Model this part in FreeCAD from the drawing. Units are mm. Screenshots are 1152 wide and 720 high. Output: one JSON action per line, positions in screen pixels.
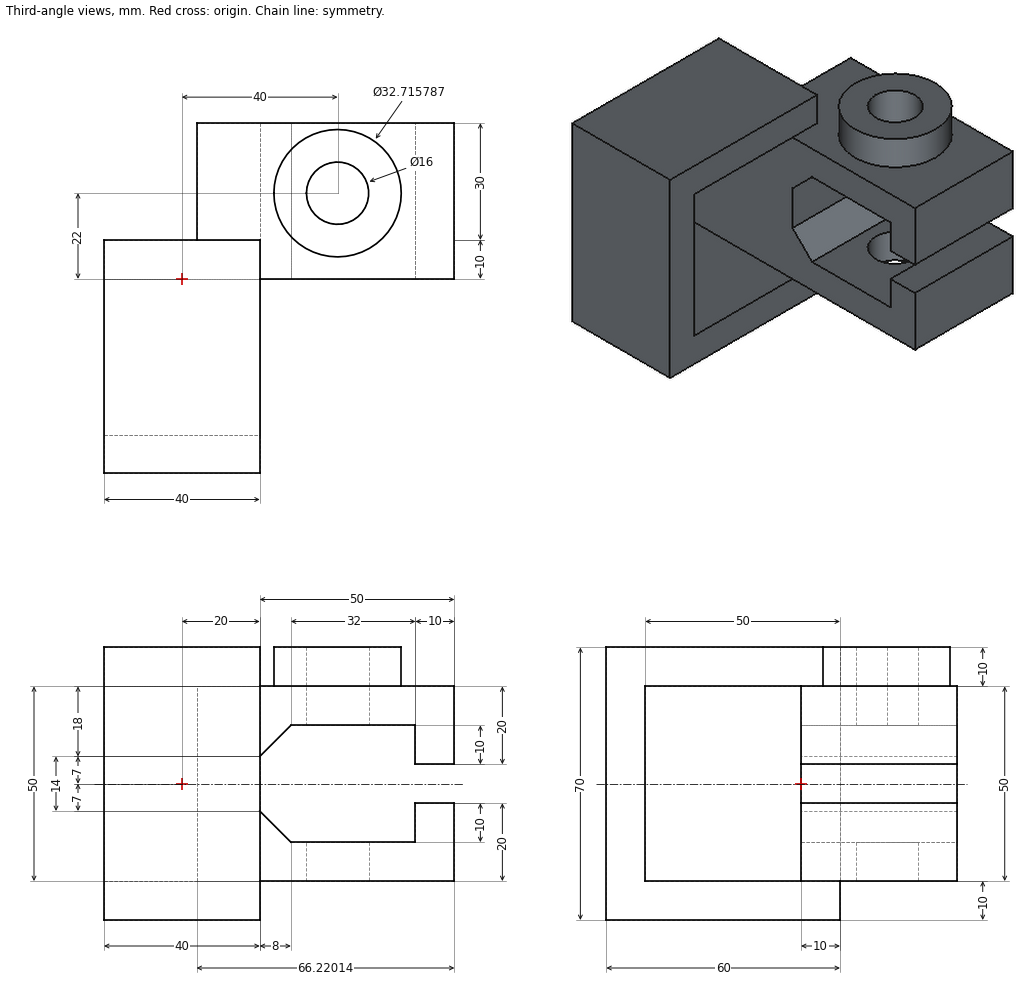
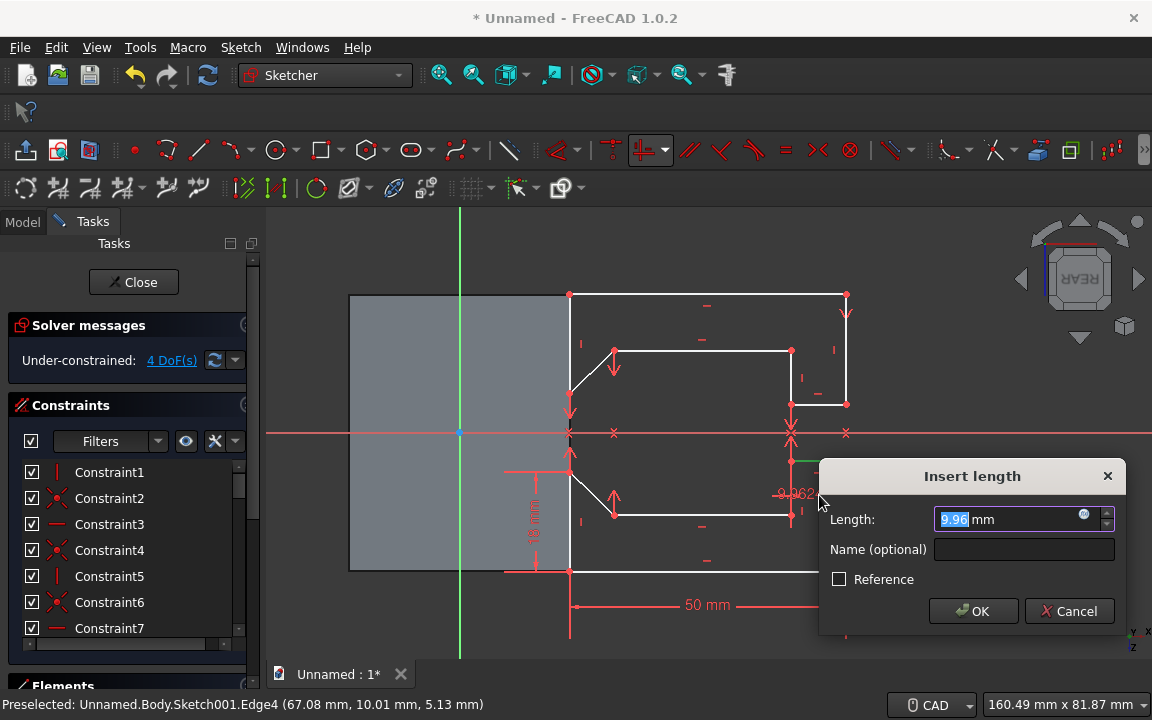
{"action": "type", "text": "10"}
{"action": "key", "text": "Return"}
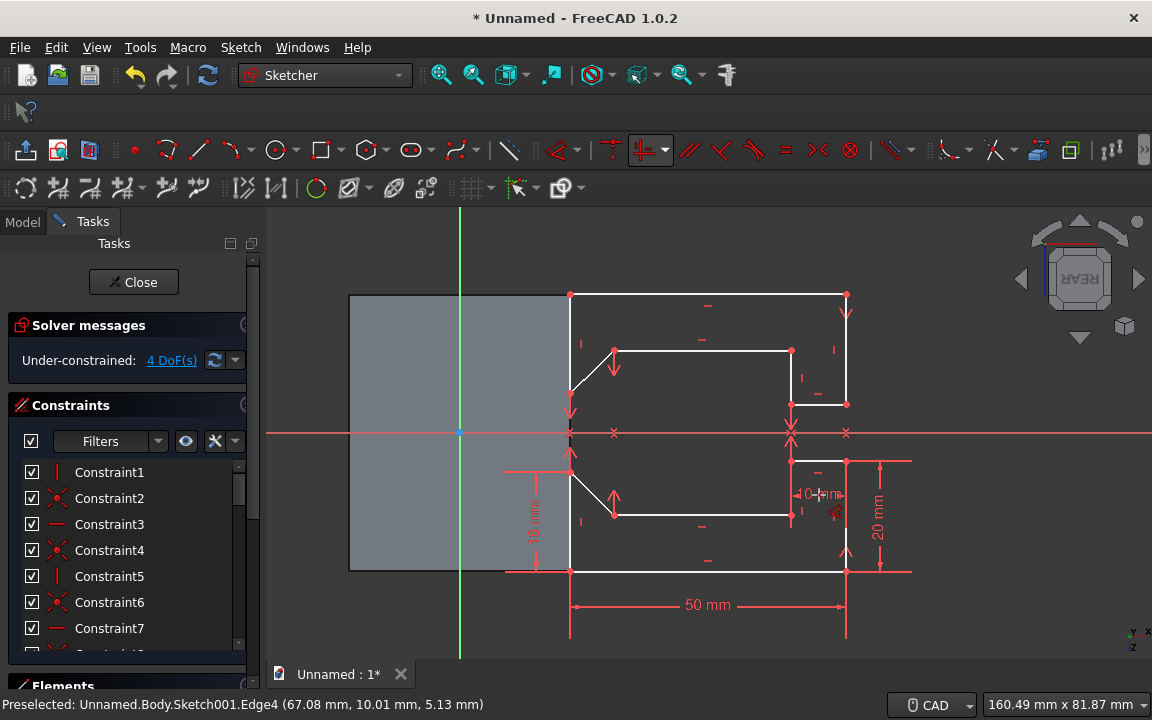
{"action": "left_click", "coordinate": [791, 477]}
{"action": "left_click", "coordinate": [757, 469]}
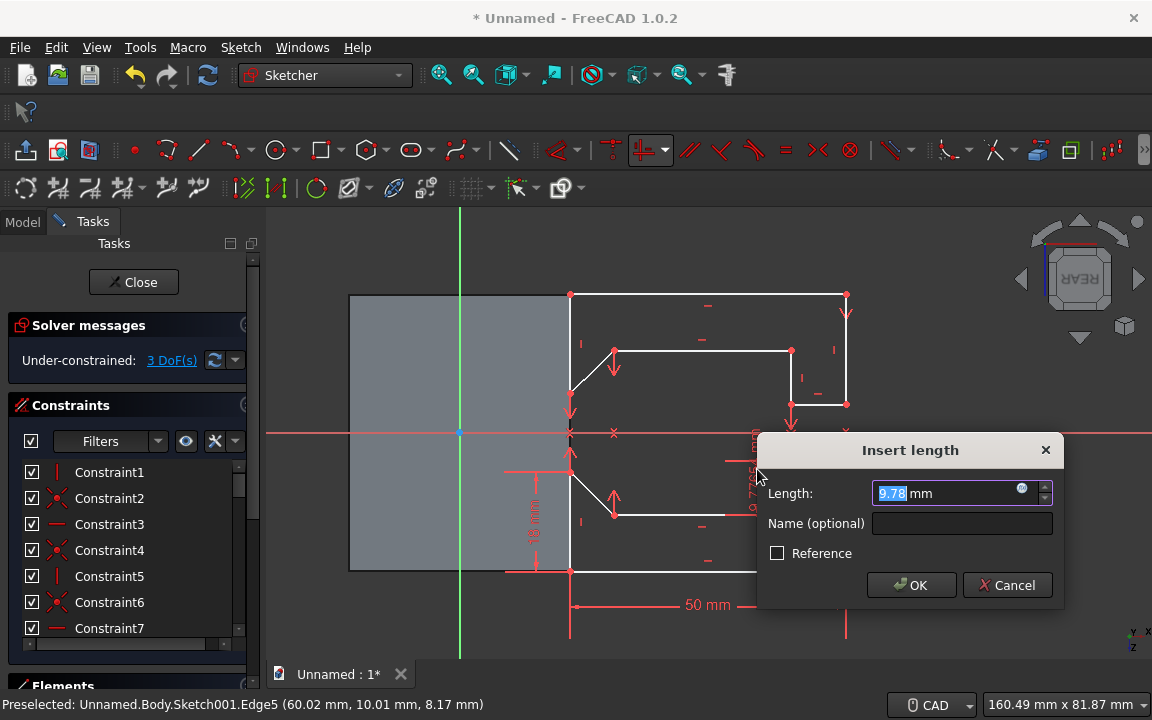
{"action": "type", "text": "10"}
{"action": "key", "text": "Return"}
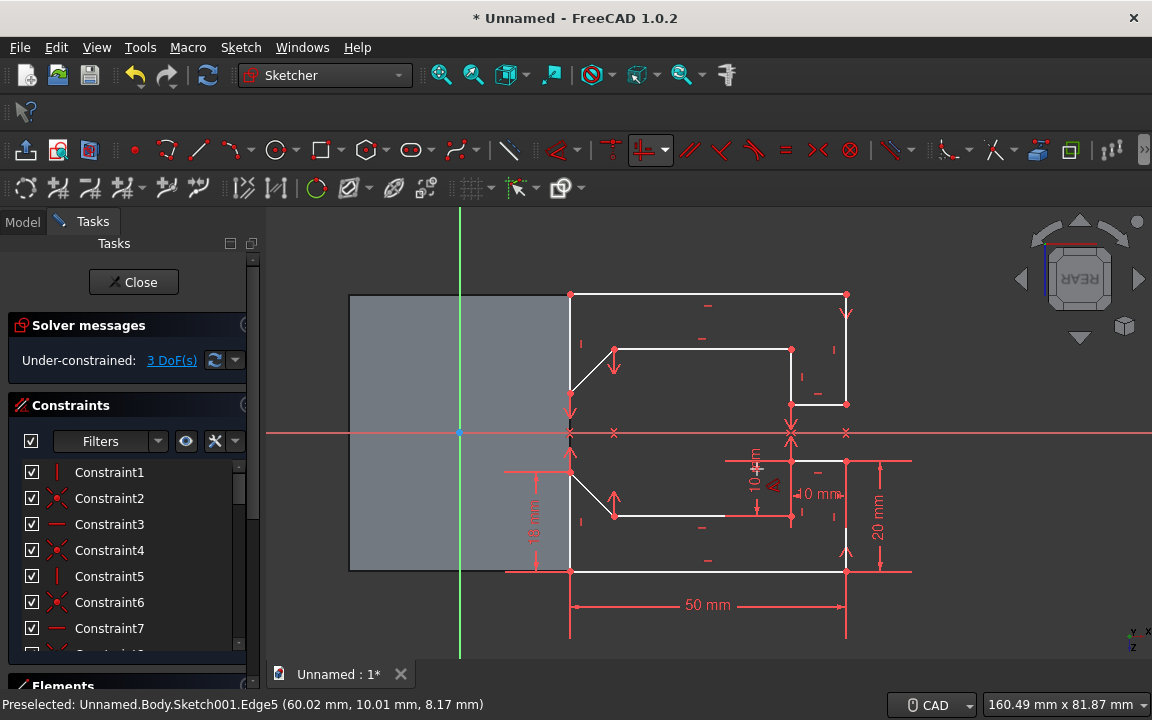
{"action": "left_click", "coordinate": [738, 516]}
{"action": "left_click", "coordinate": [703, 550]}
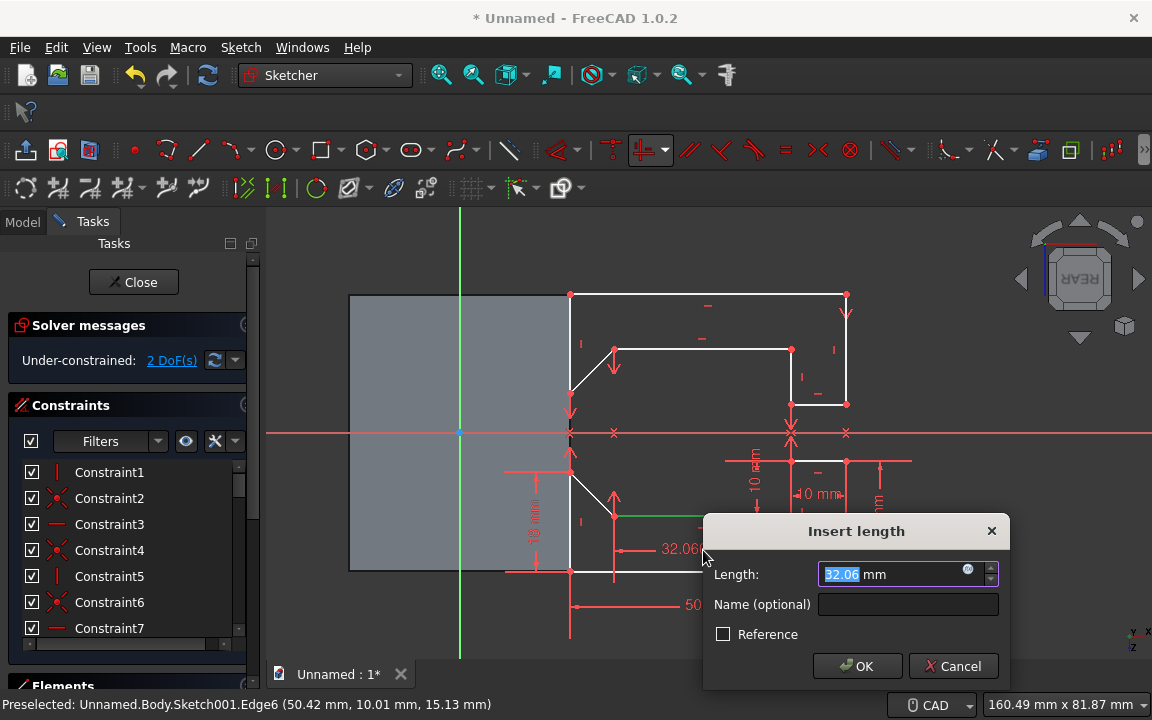
{"action": "type", "text": "32"}
{"action": "key", "text": "Return"}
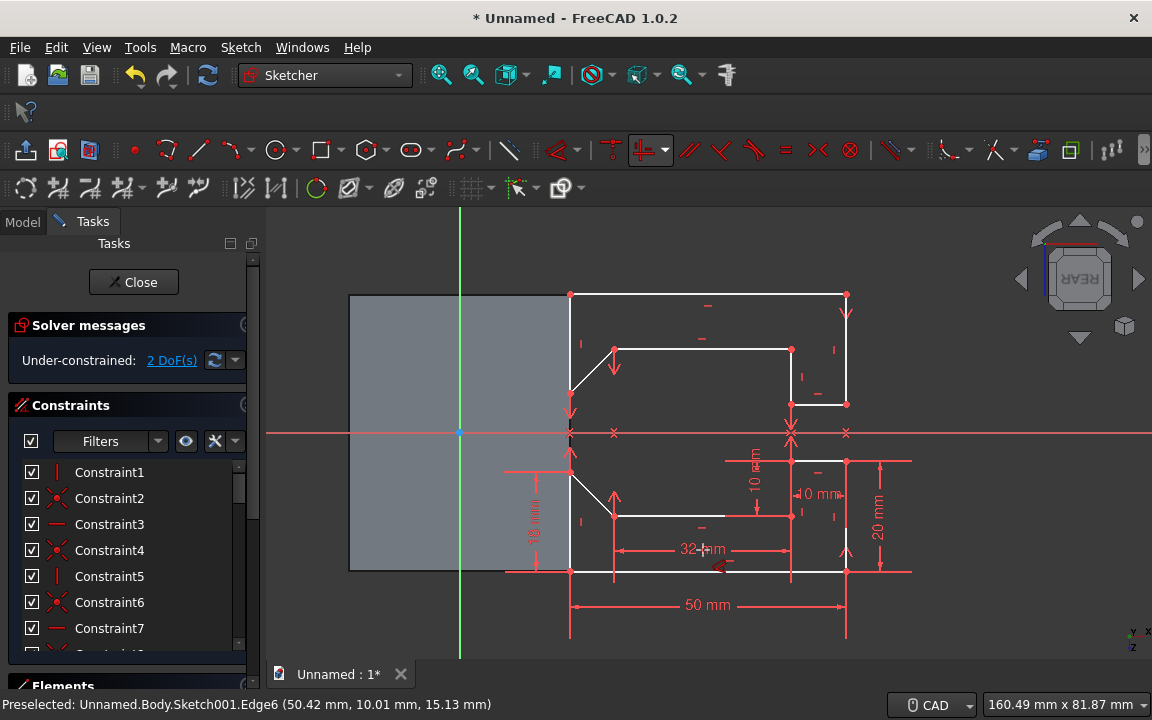
{"action": "left_click", "coordinate": [570, 472]}
{"action": "left_click", "coordinate": [426, 453]}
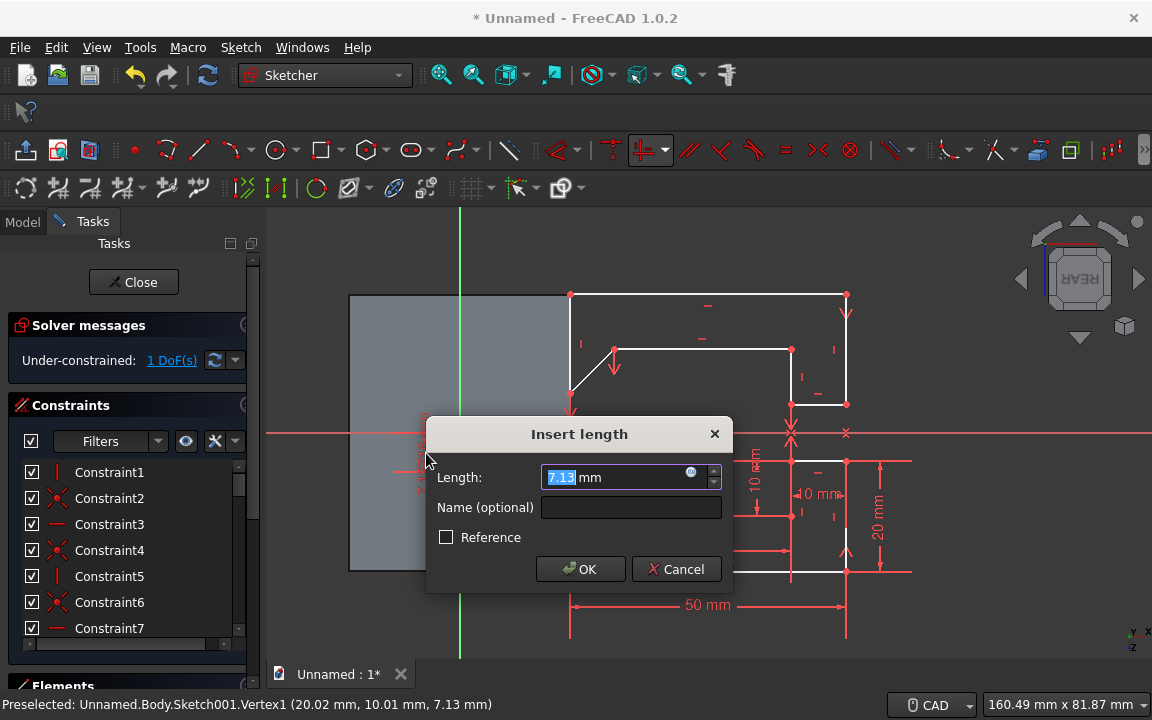
{"action": "type", "text": "7"}
{"action": "key", "text": "Return"}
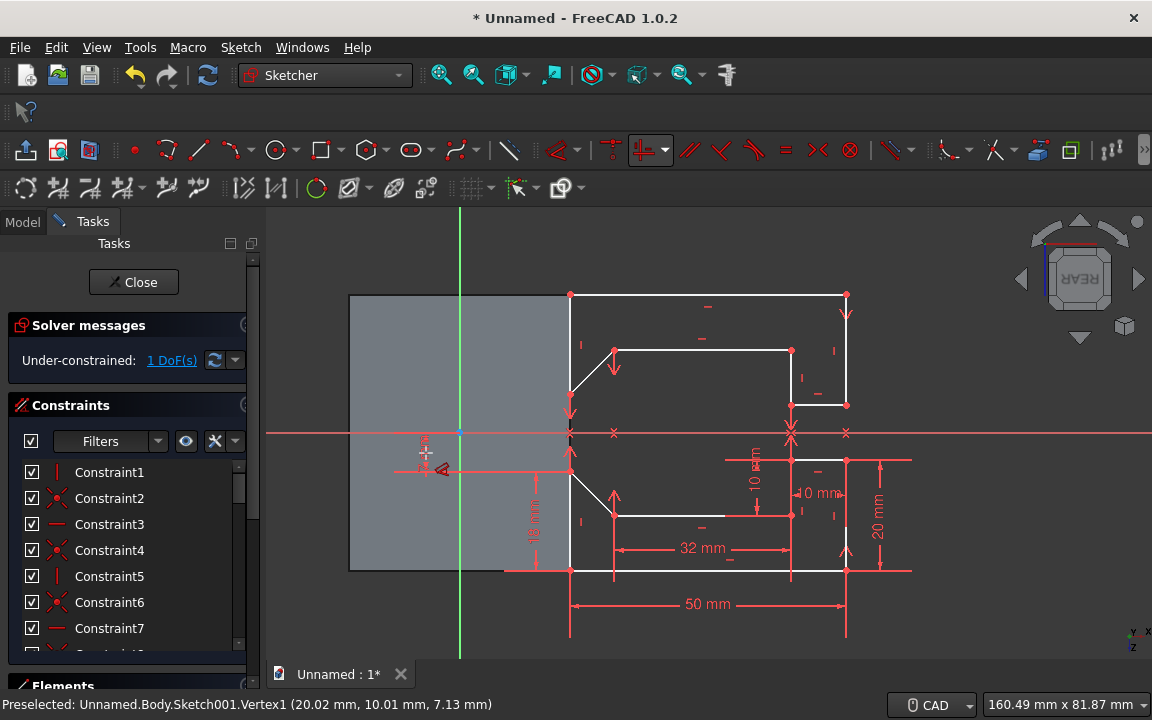
{"action": "left_click", "coordinate": [570, 472]}
{"action": "left_click", "coordinate": [515, 399]}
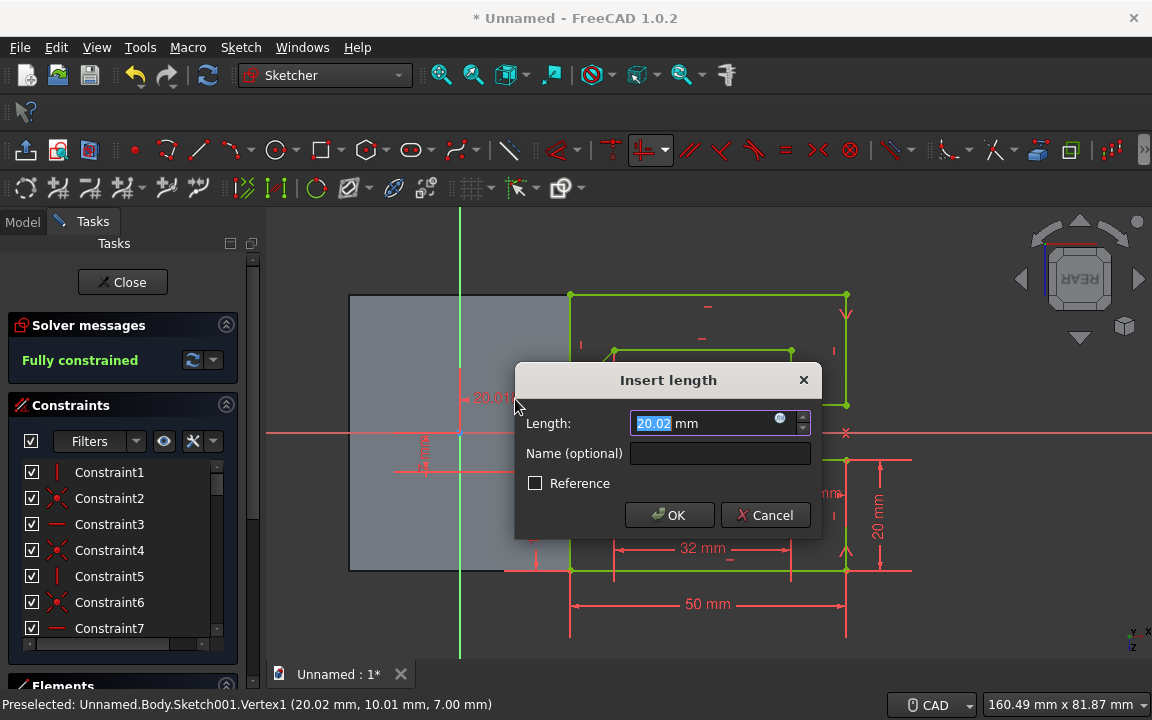
{"action": "type", "text": "20"}
{"action": "key", "text": "Return"}
{"action": "key", "text": "Escape"}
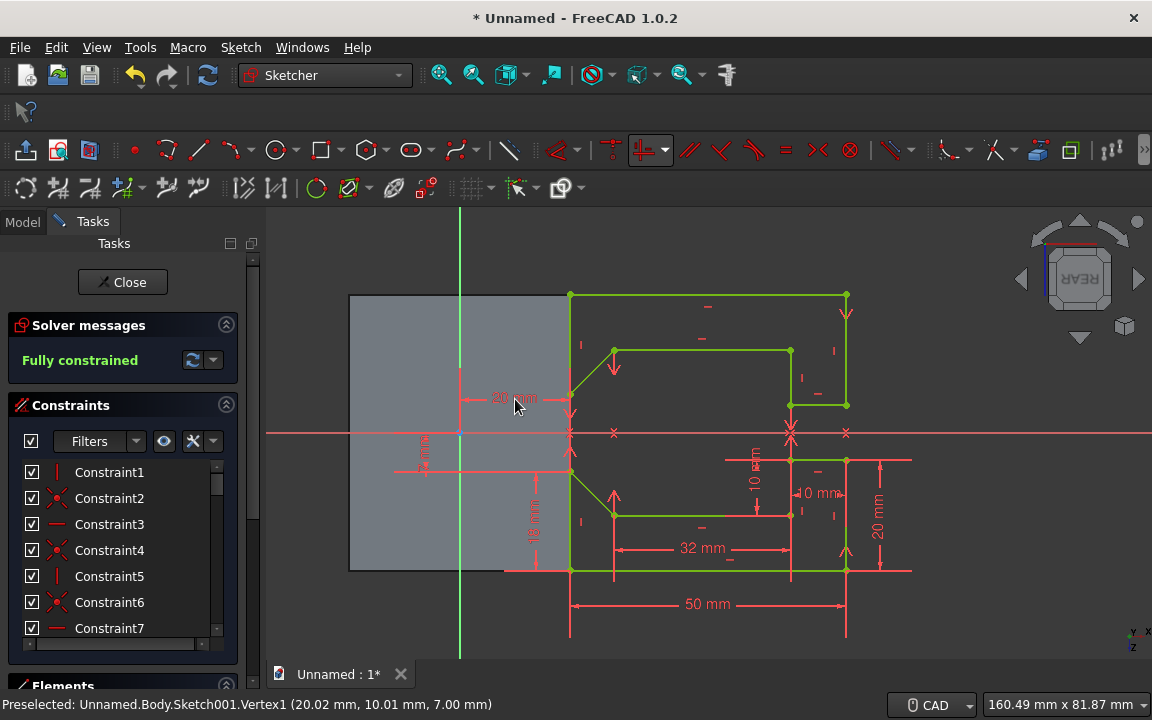
{"action": "left_click", "coordinate": [123, 282]}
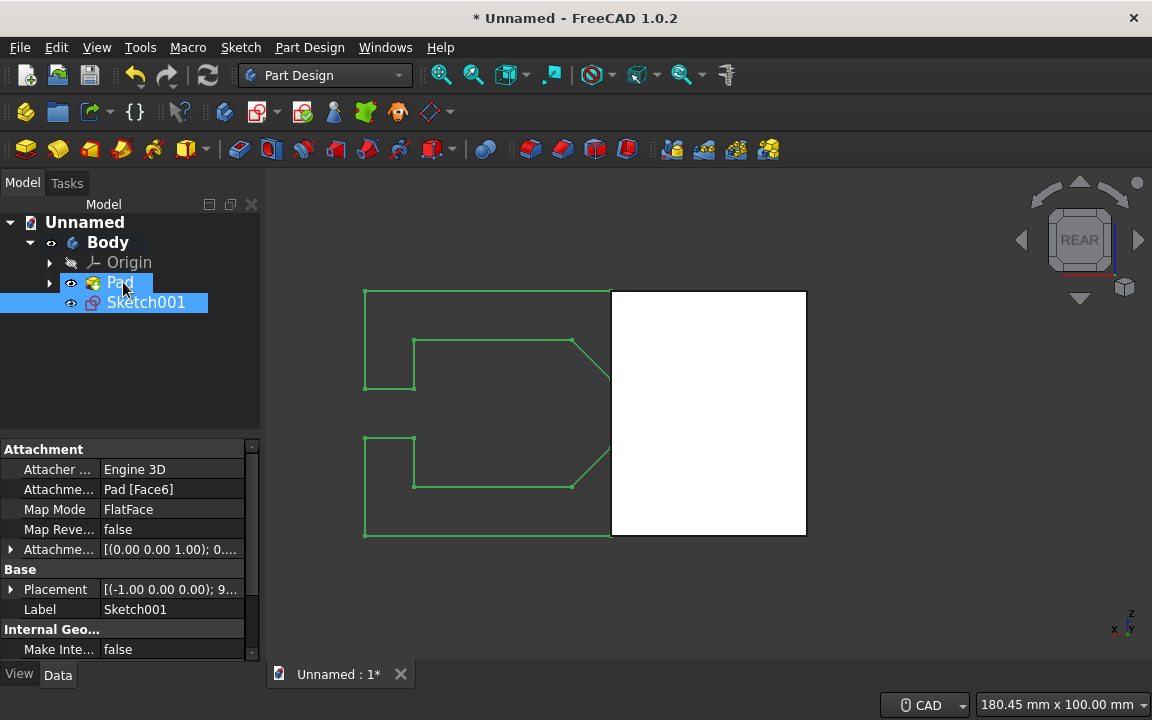
{"action": "left_click", "coordinate": [26, 150]}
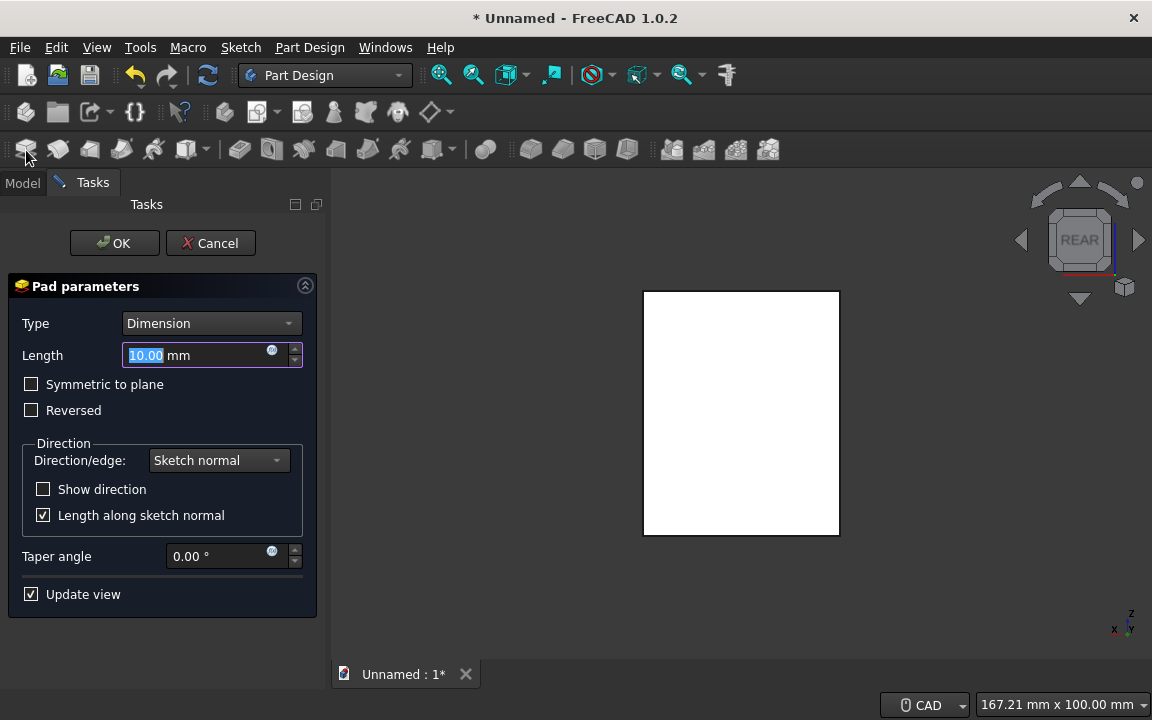
{"action": "type", "text": "10"}
{"action": "key", "text": "Tab"}